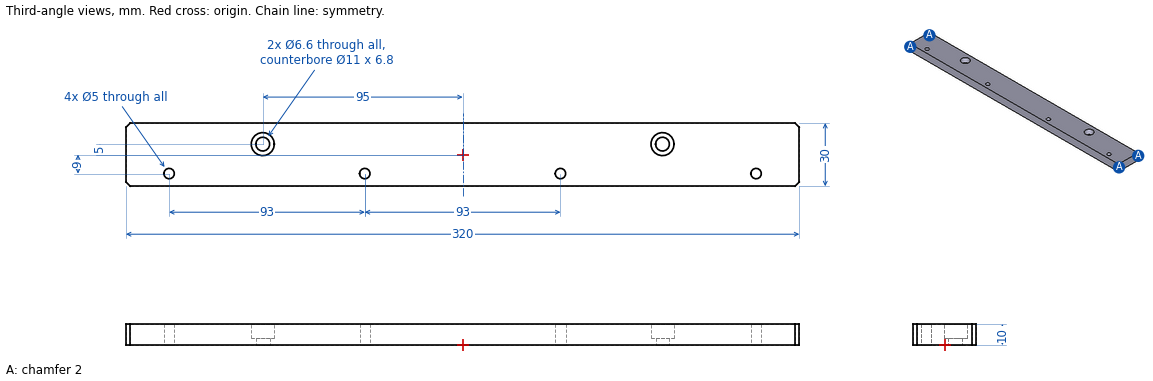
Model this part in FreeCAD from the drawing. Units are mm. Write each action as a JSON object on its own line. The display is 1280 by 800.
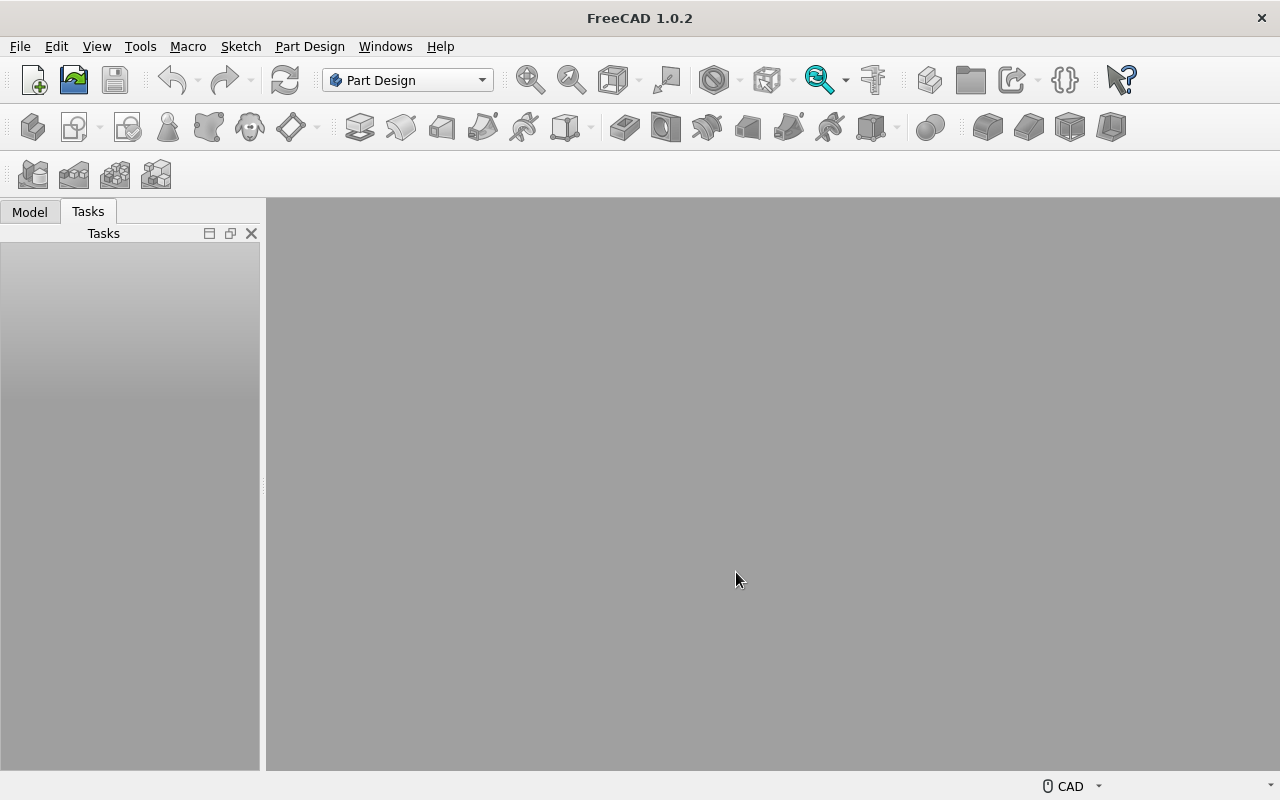
{"action": "left_click", "coordinate": [33, 80]}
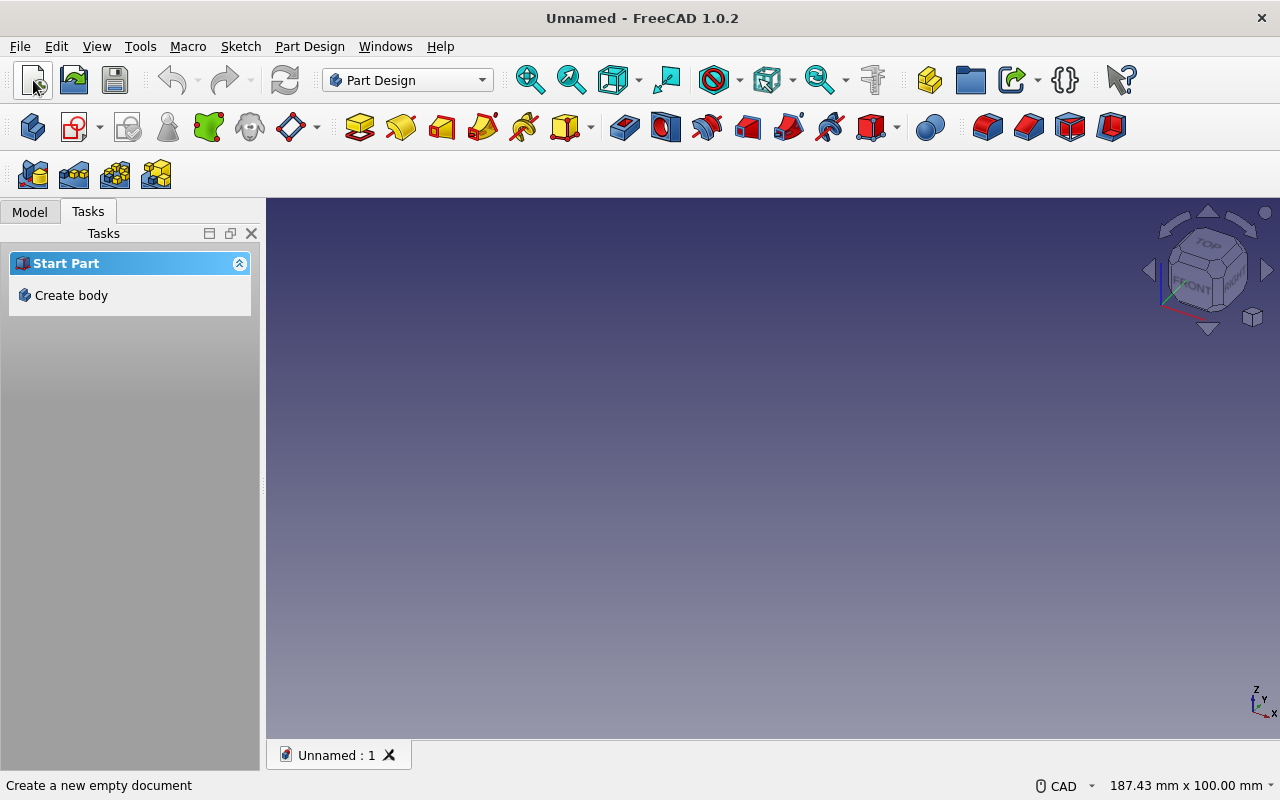
{"action": "left_click", "coordinate": [74, 128]}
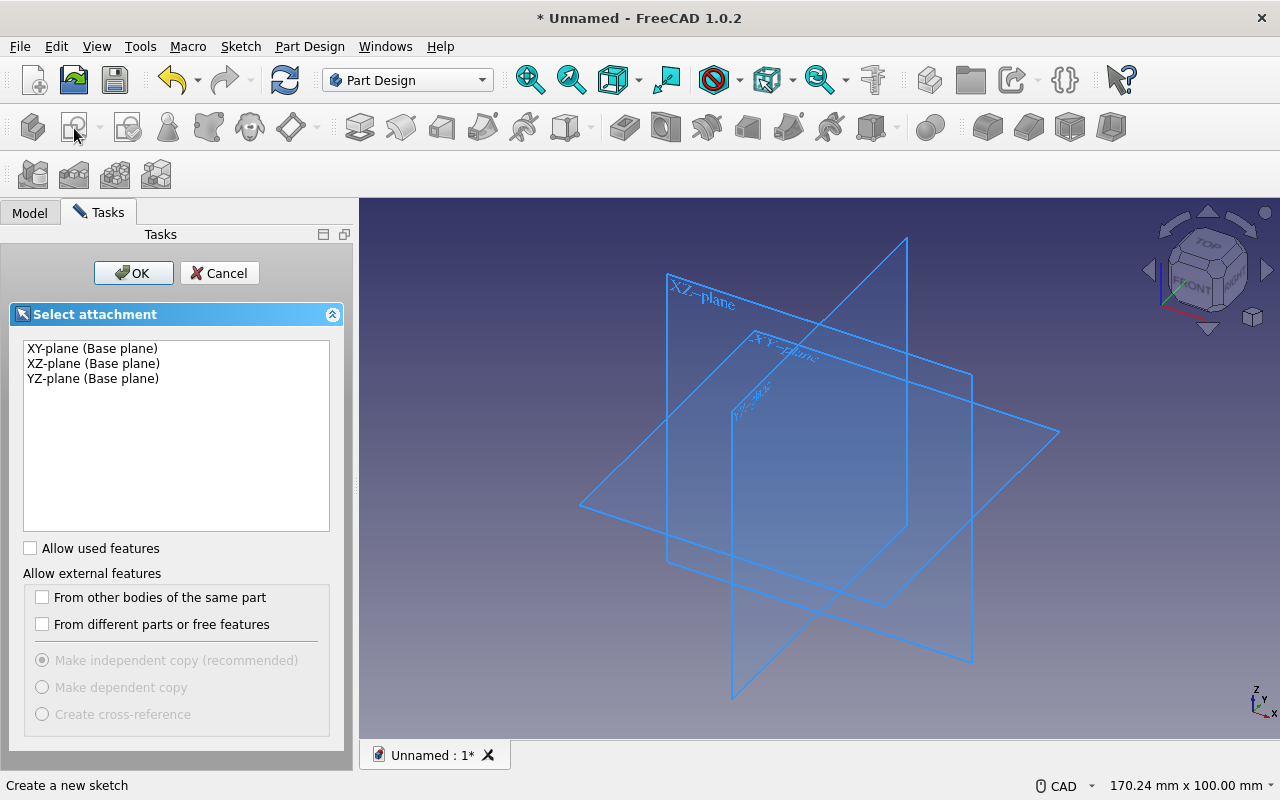
{"action": "left_click", "coordinate": [84, 348]}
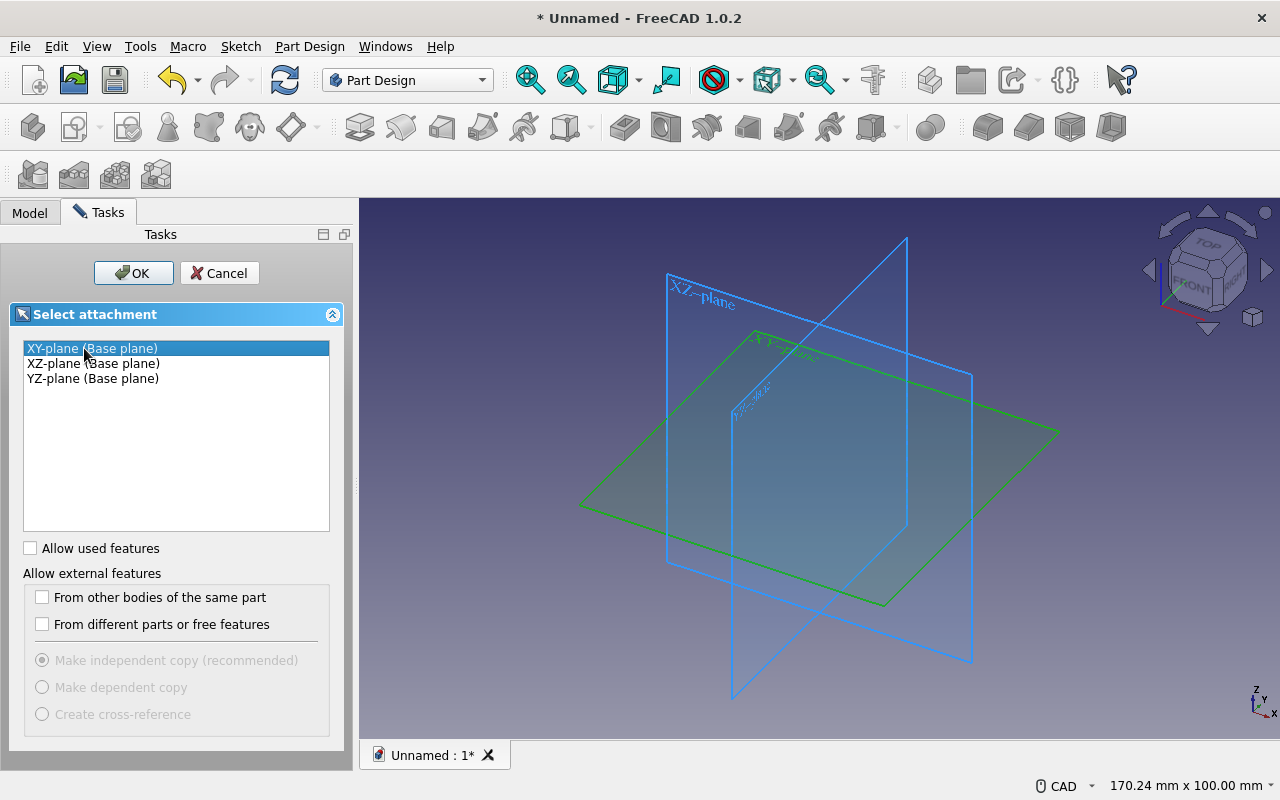
{"action": "left_click", "coordinate": [134, 273]}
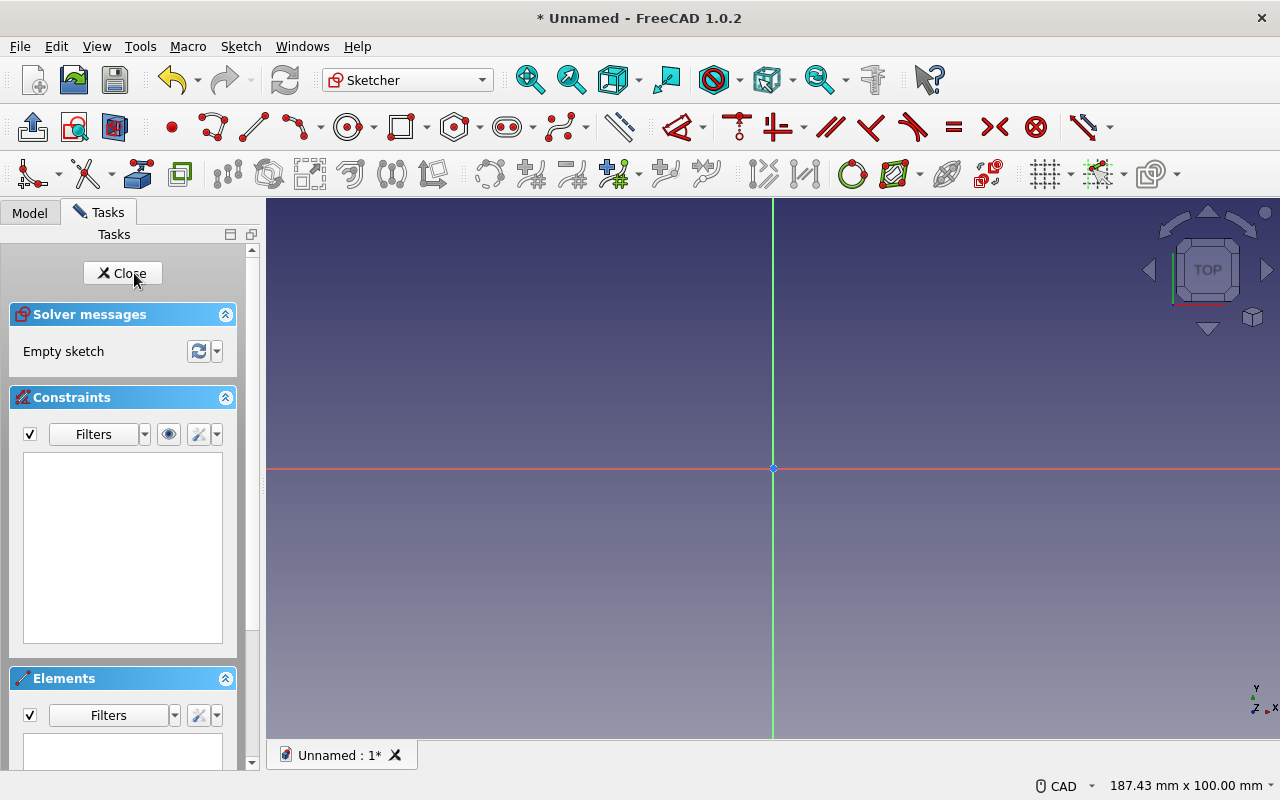
{"action": "scroll", "coordinate": [665, 469], "scroll_direction": "down", "scroll_amount": 5}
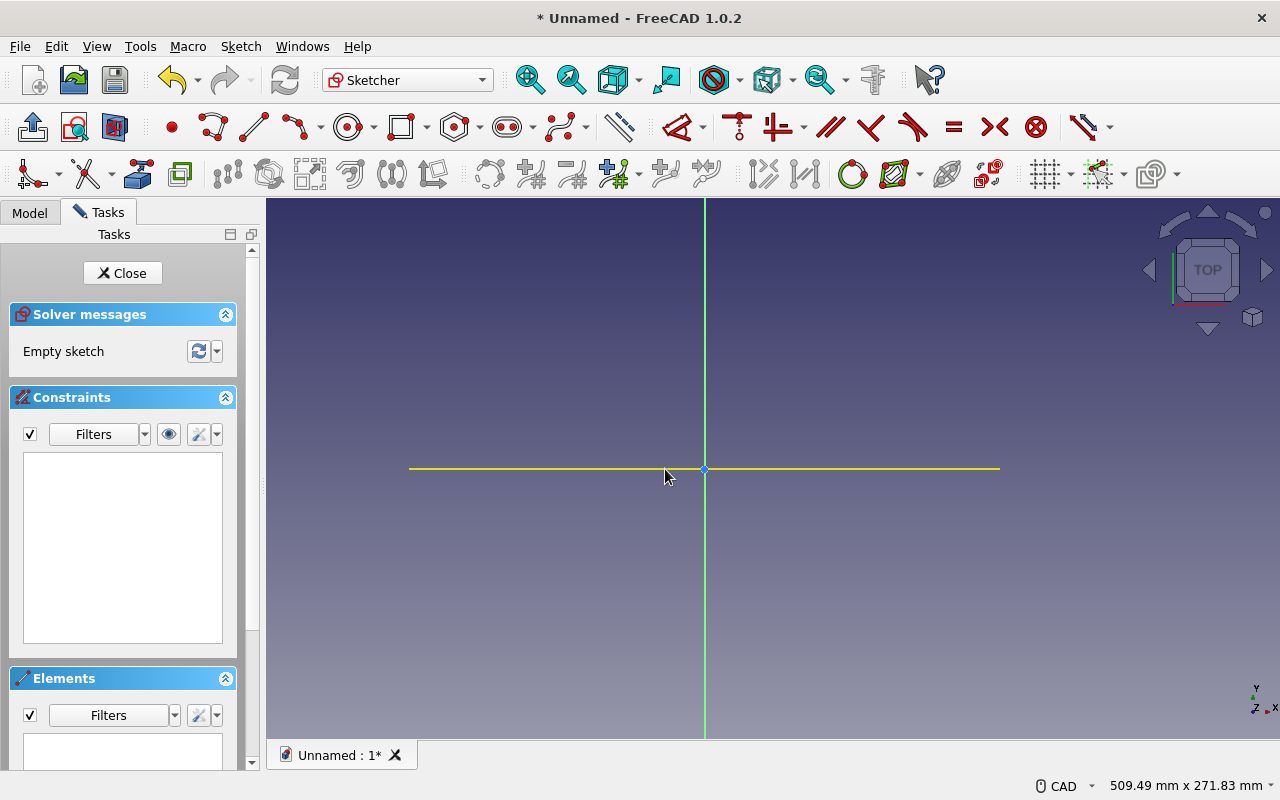
{"action": "left_click", "coordinate": [426, 128]}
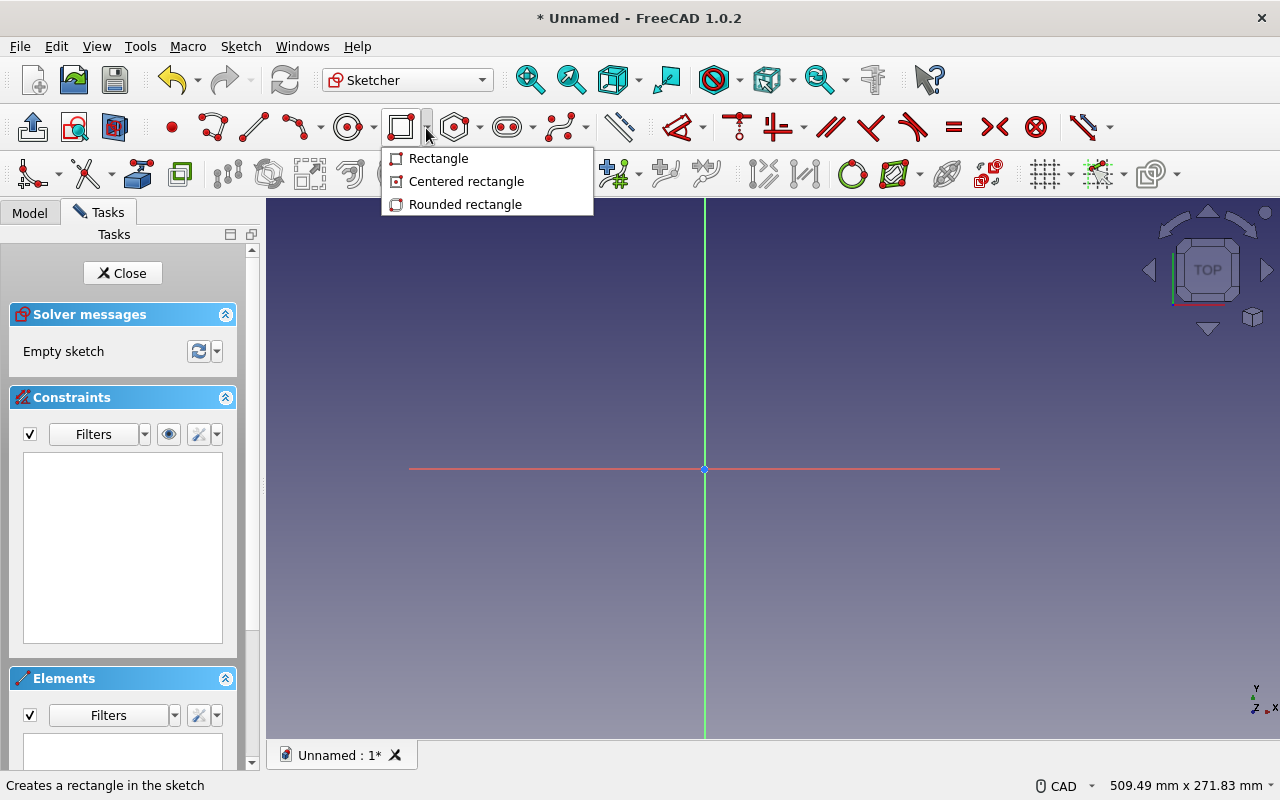
{"action": "left_click", "coordinate": [488, 182]}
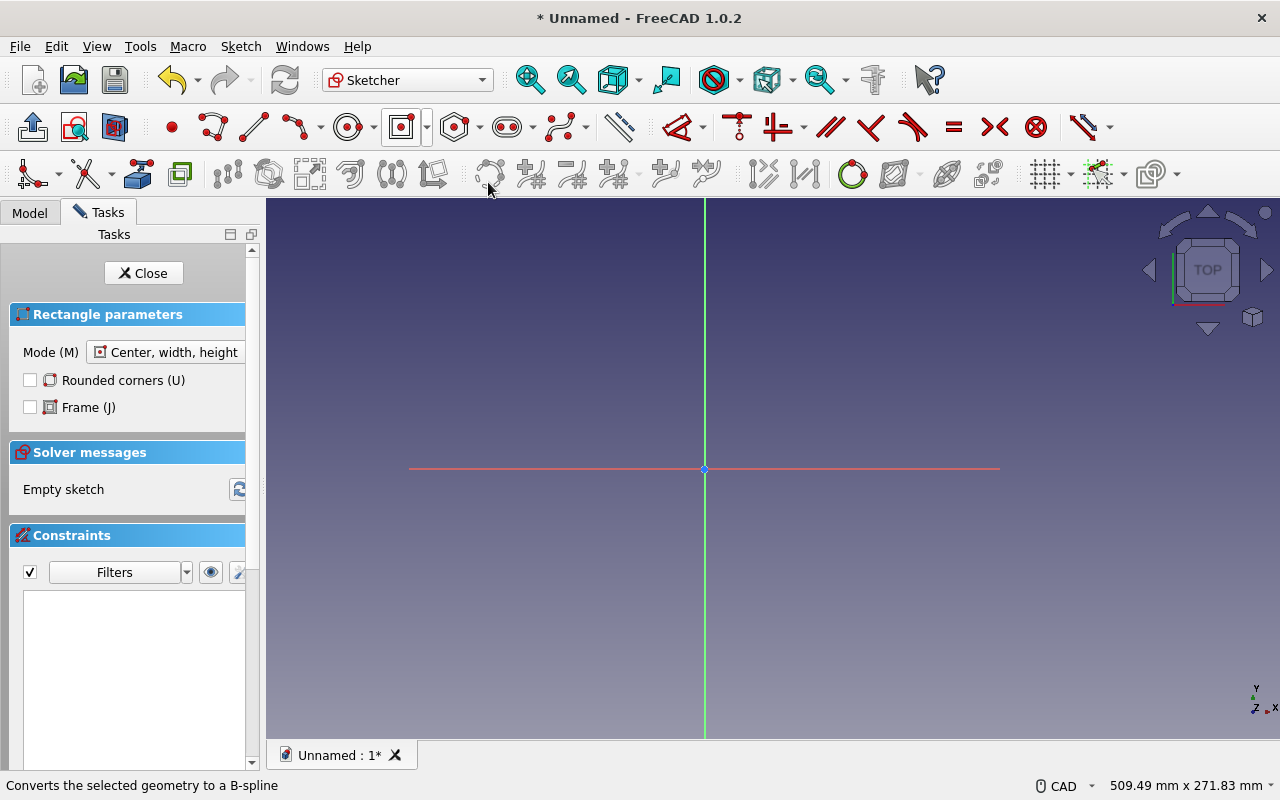
{"action": "left_click", "coordinate": [705, 469]}
{"action": "left_click", "coordinate": [1023, 439]}
{"action": "key", "text": "Escape"}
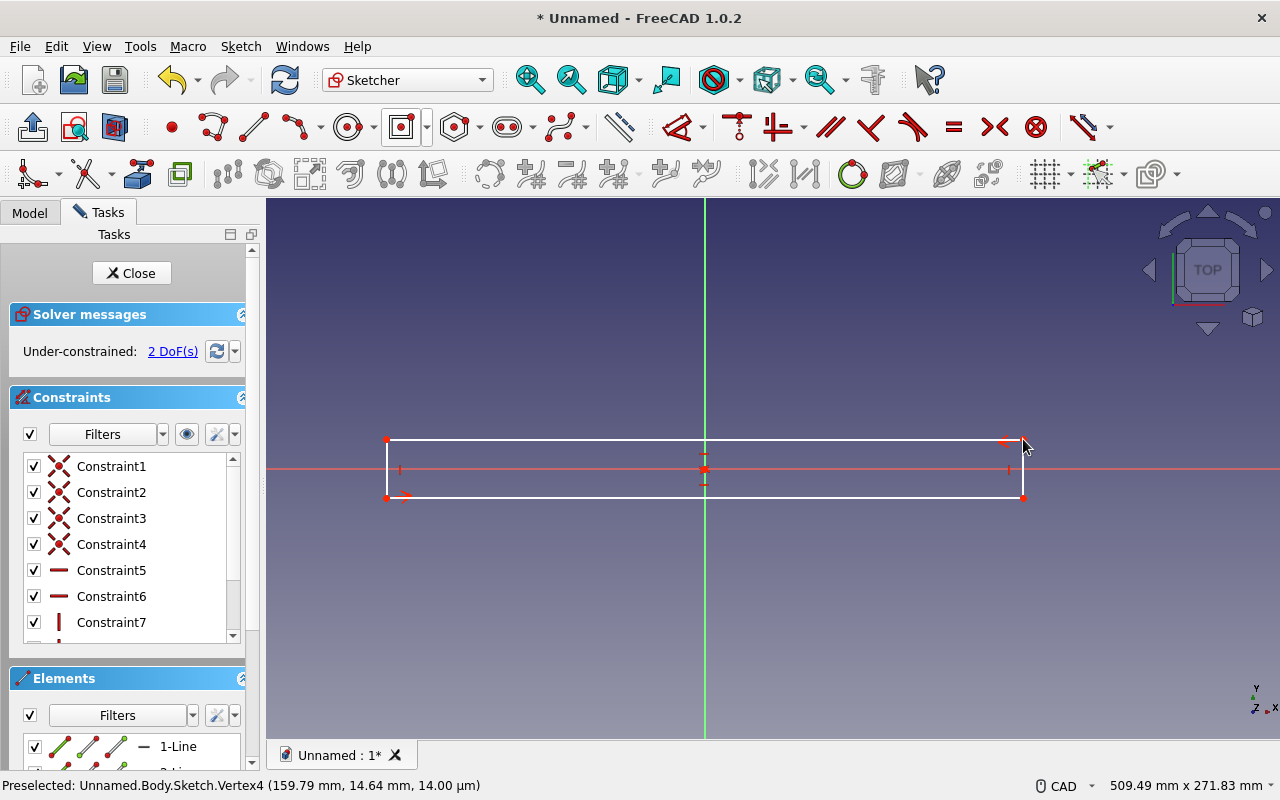
{"action": "left_click", "coordinate": [676, 128]}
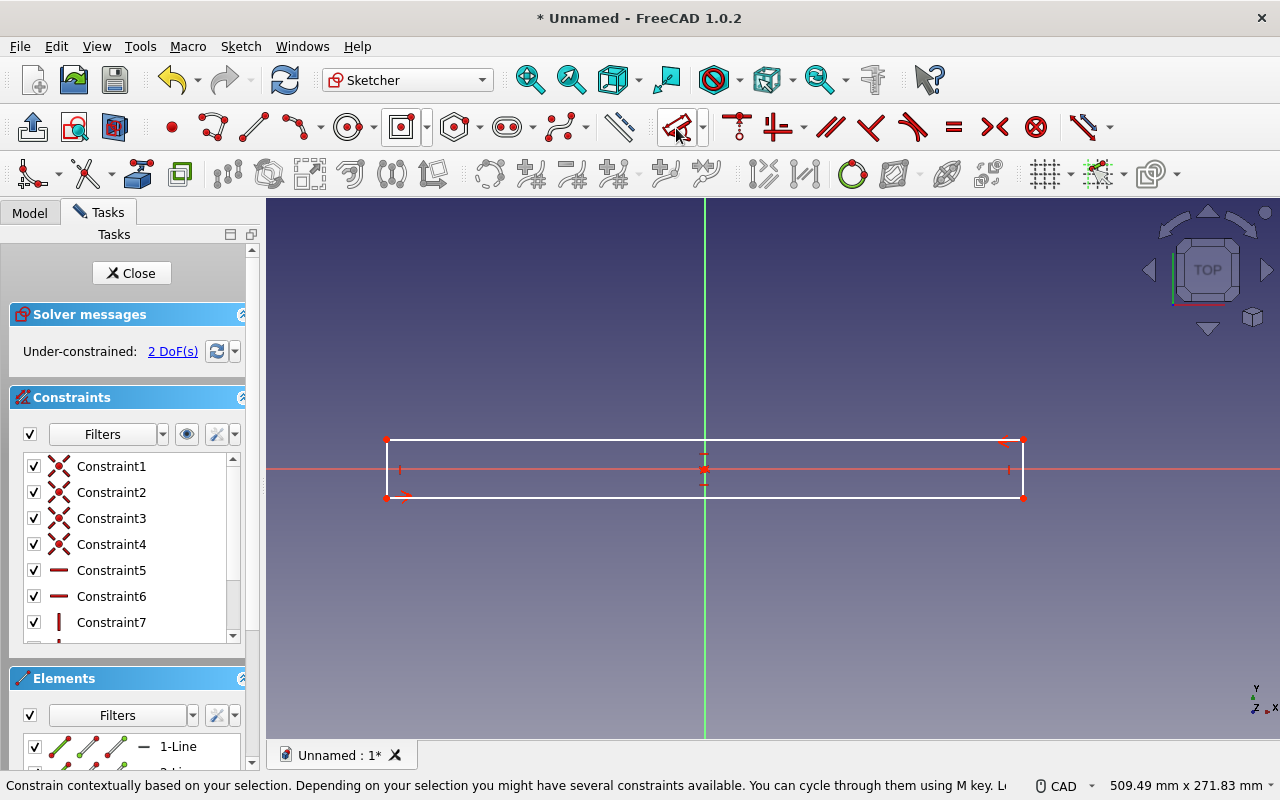
{"action": "left_click", "coordinate": [1023, 481]}
{"action": "left_click", "coordinate": [1057, 456]}